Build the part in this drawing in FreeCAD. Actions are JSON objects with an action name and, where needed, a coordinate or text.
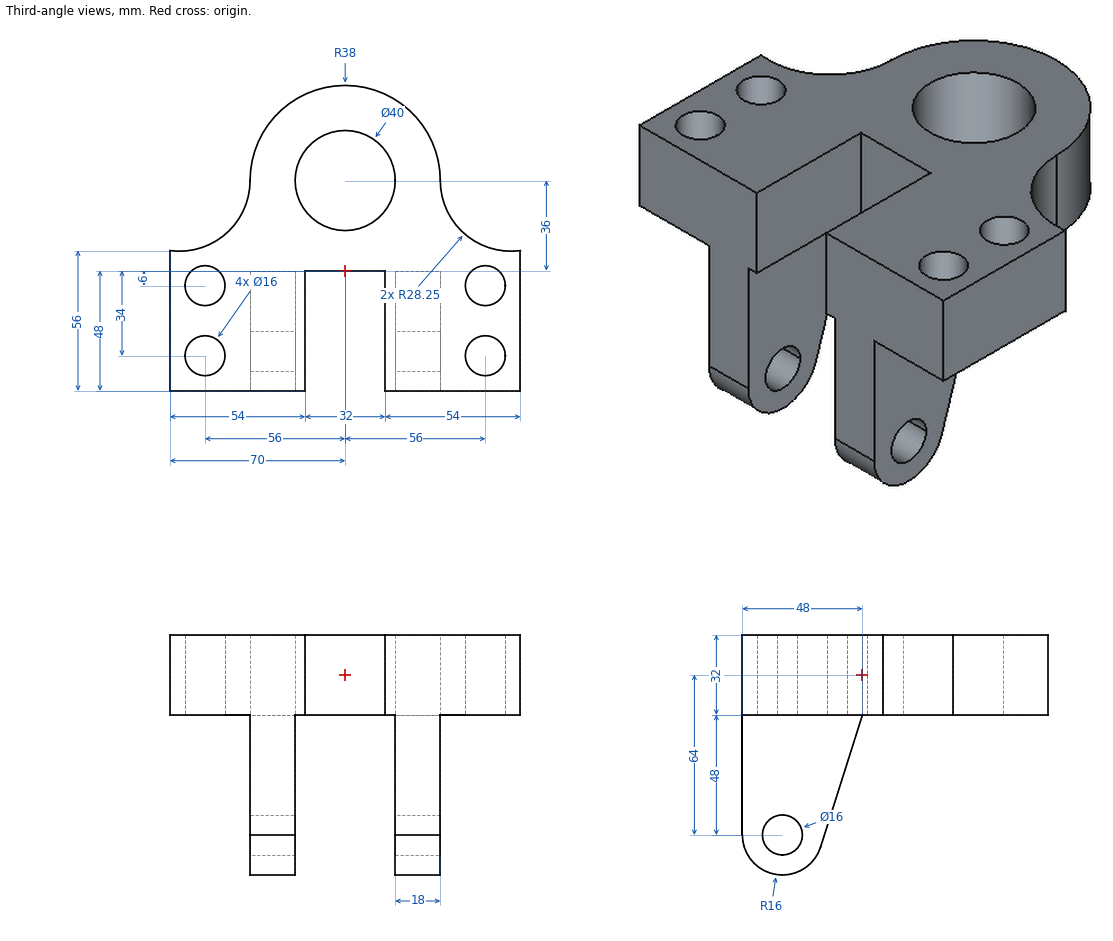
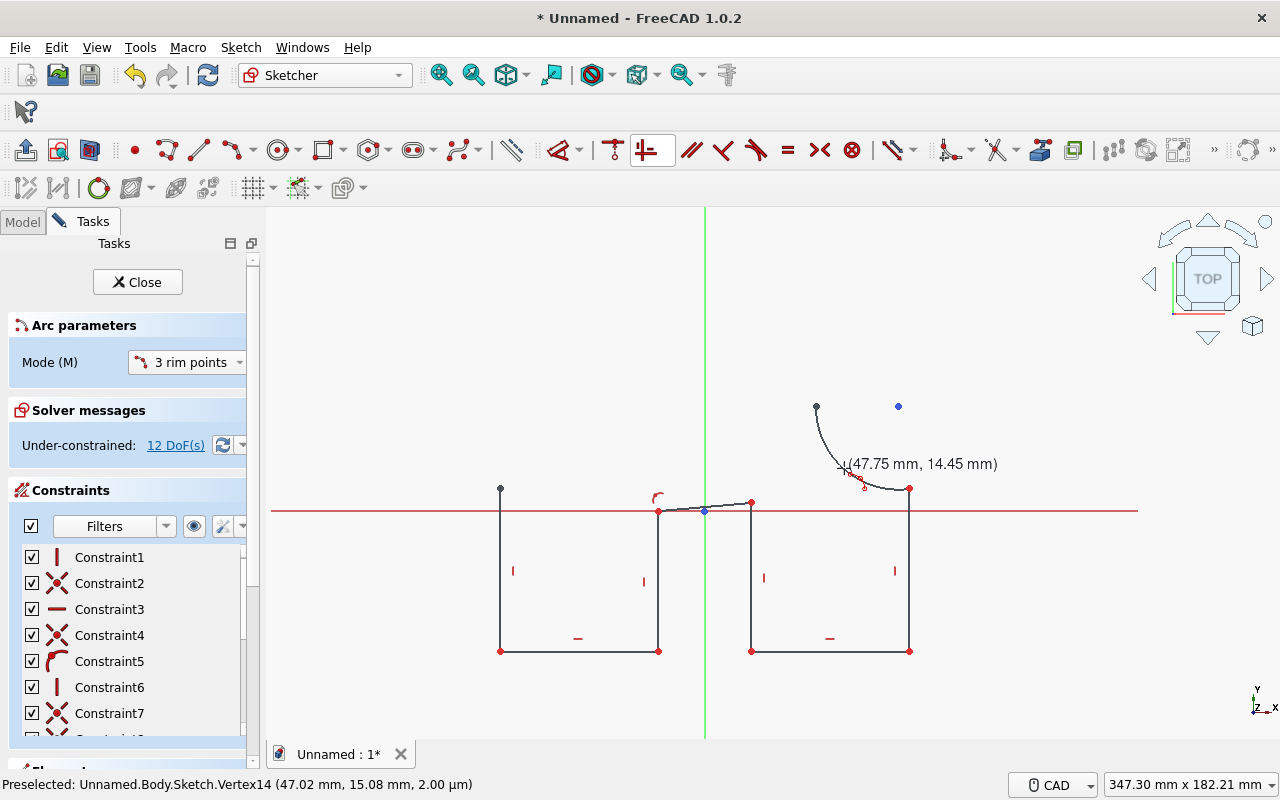
{"action": "left_click", "coordinate": [816, 407]}
{"action": "left_click", "coordinate": [594, 406]}
{"action": "left_click", "coordinate": [739, 301]}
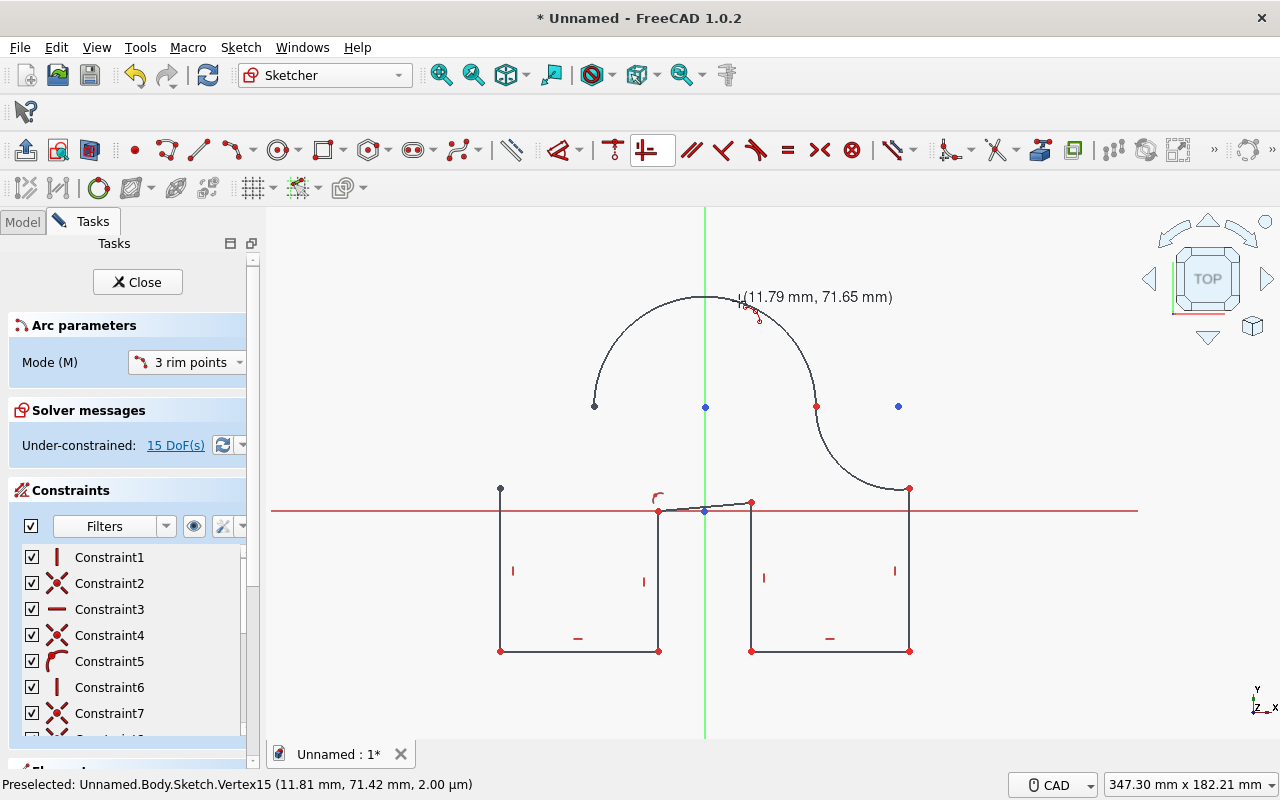
{"action": "left_click", "coordinate": [594, 407]}
{"action": "left_click", "coordinate": [500, 489]}
{"action": "left_click", "coordinate": [565, 468]}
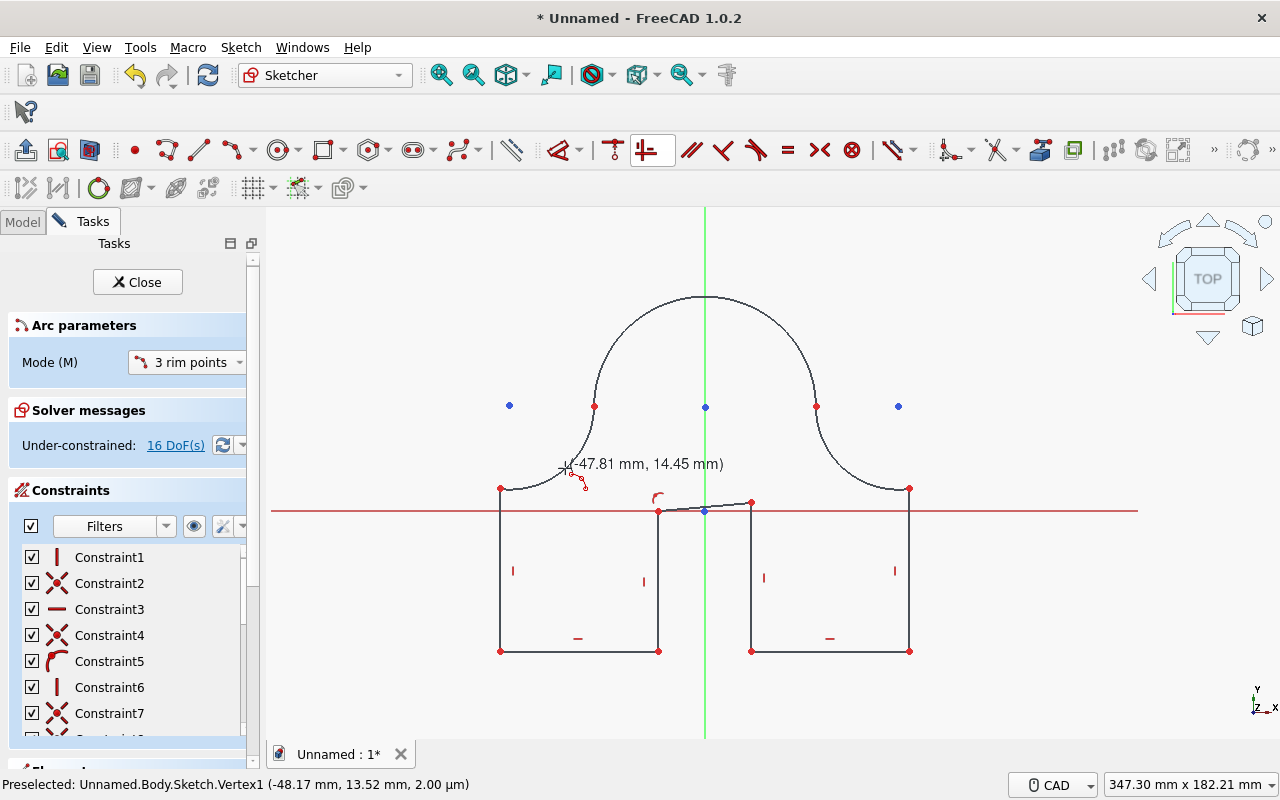
{"action": "left_click", "coordinate": [278, 150]}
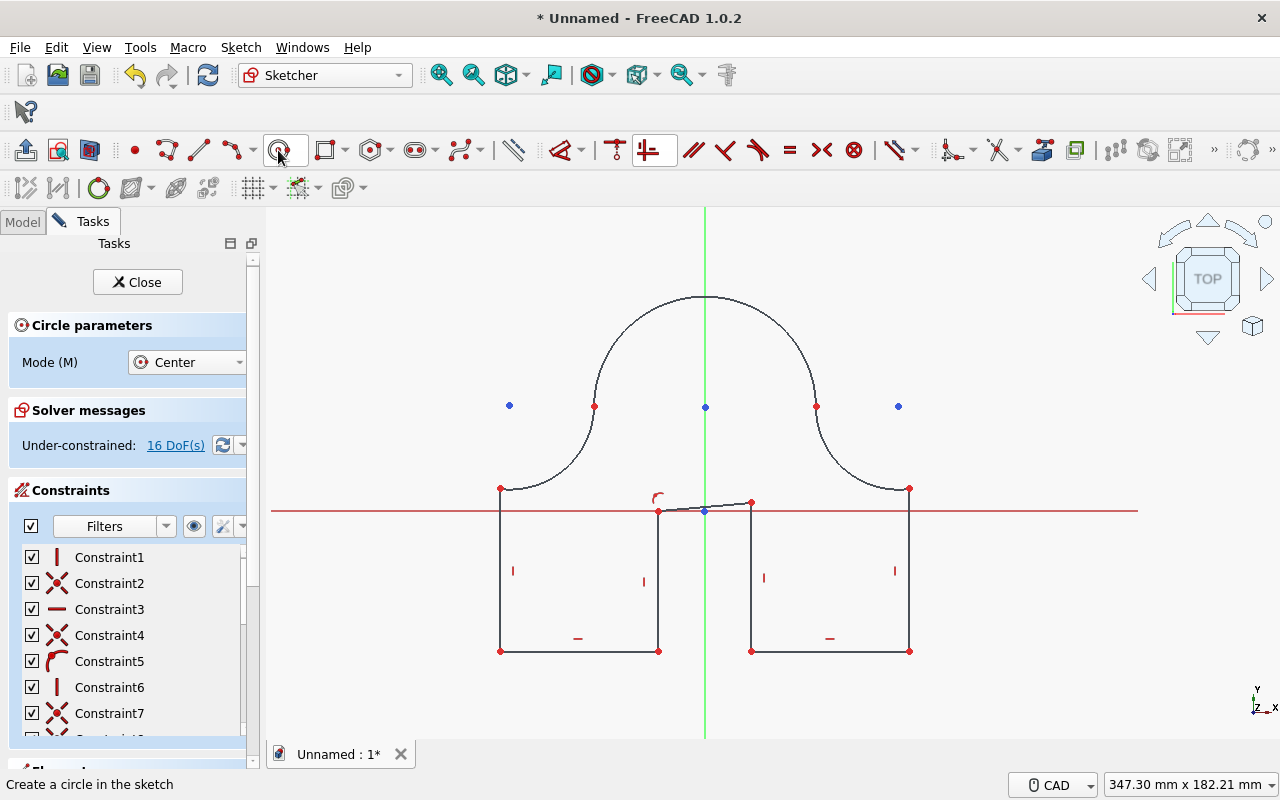
{"action": "left_click", "coordinate": [541, 610]}
{"action": "mouse_move", "coordinate": [558, 594]}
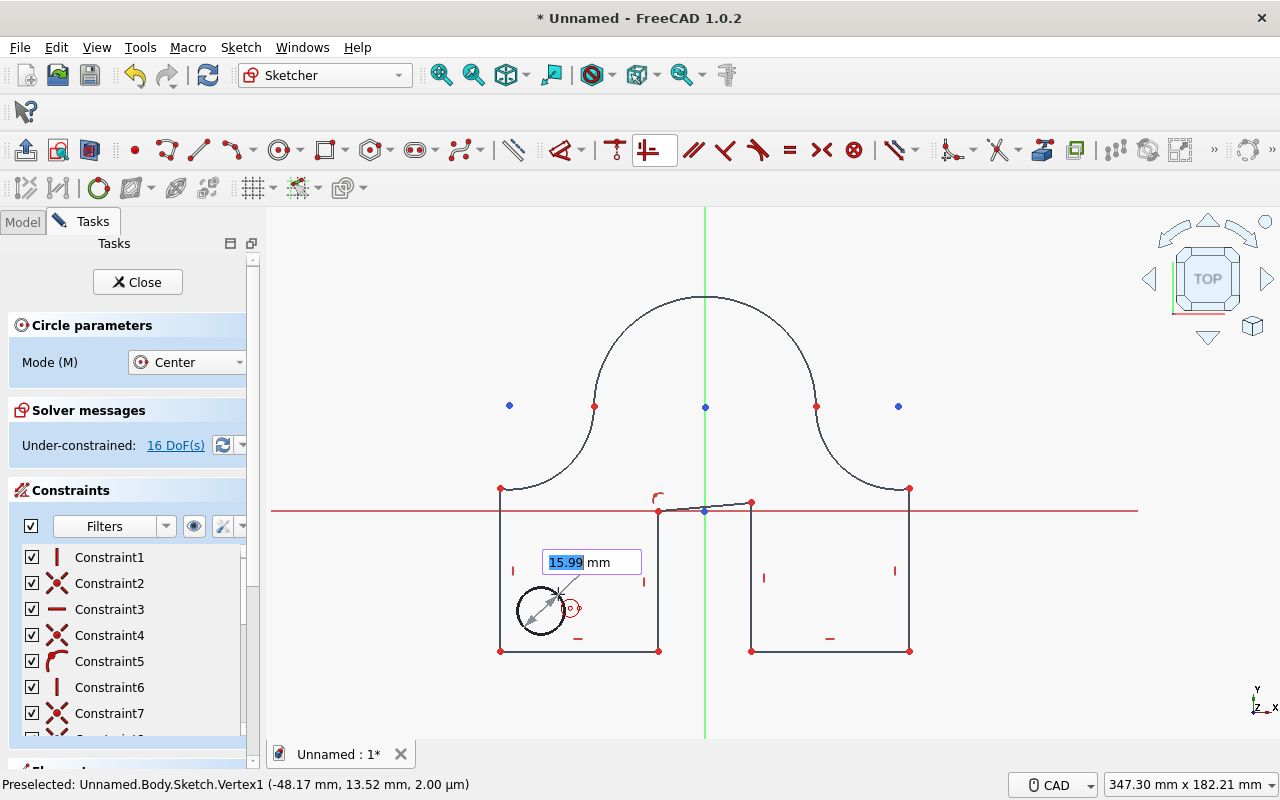
{"action": "type", "text": "16"}
{"action": "key", "text": "Return"}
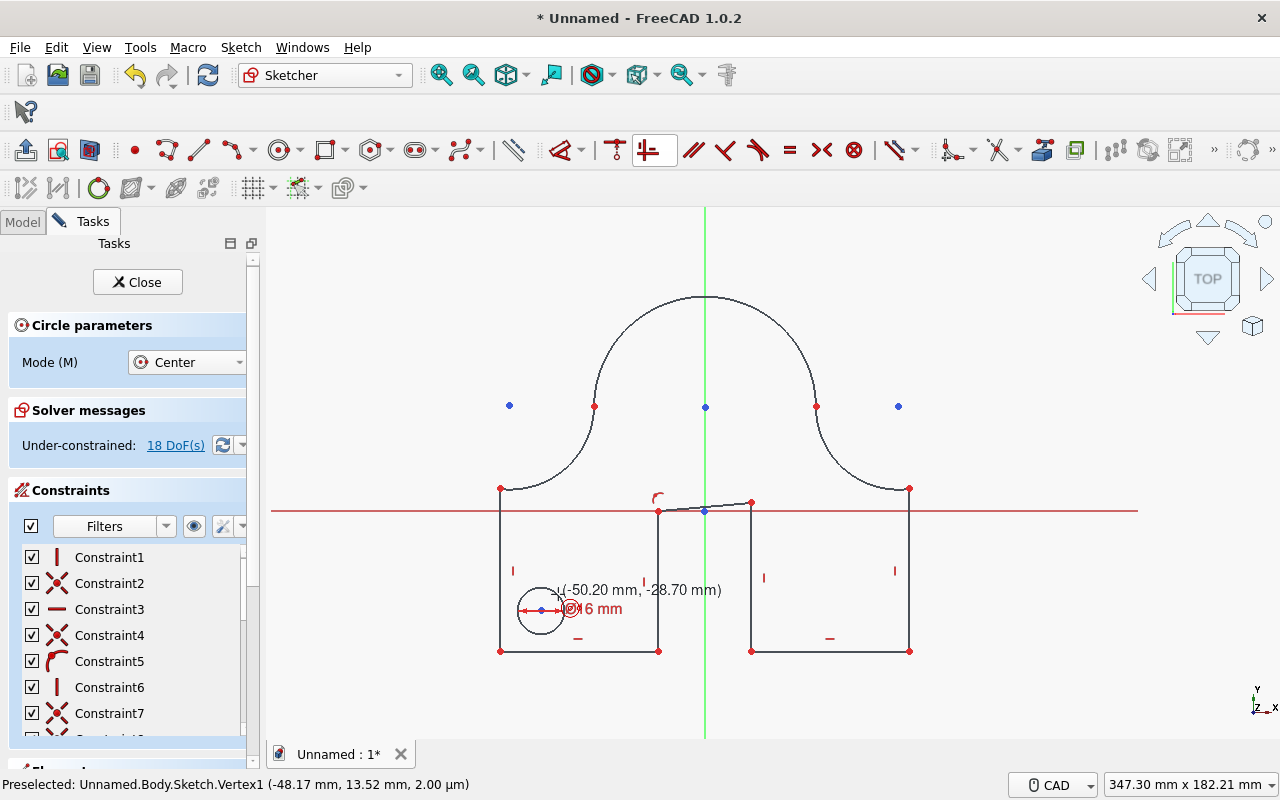
{"action": "left_click", "coordinate": [541, 529]}
{"action": "mouse_move", "coordinate": [558, 545]}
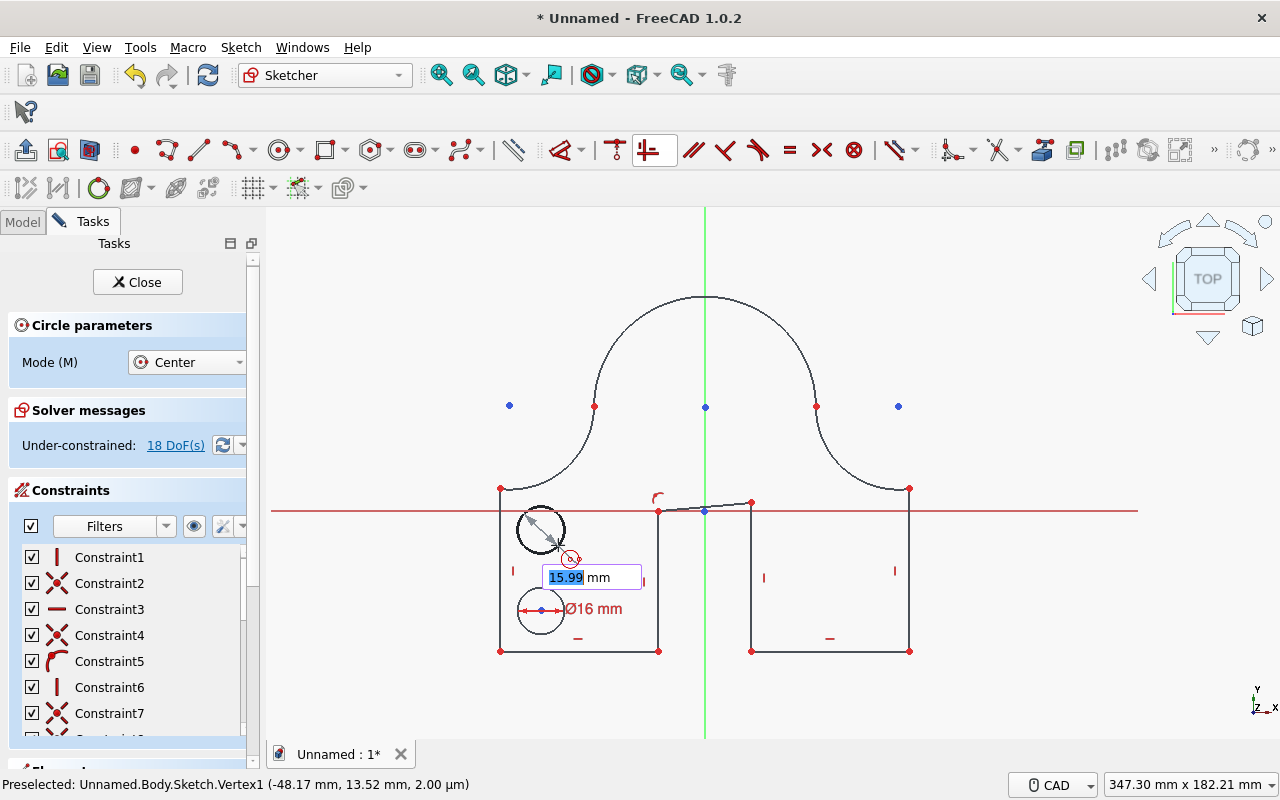
{"action": "type", "text": "16"}
{"action": "key", "text": "Return"}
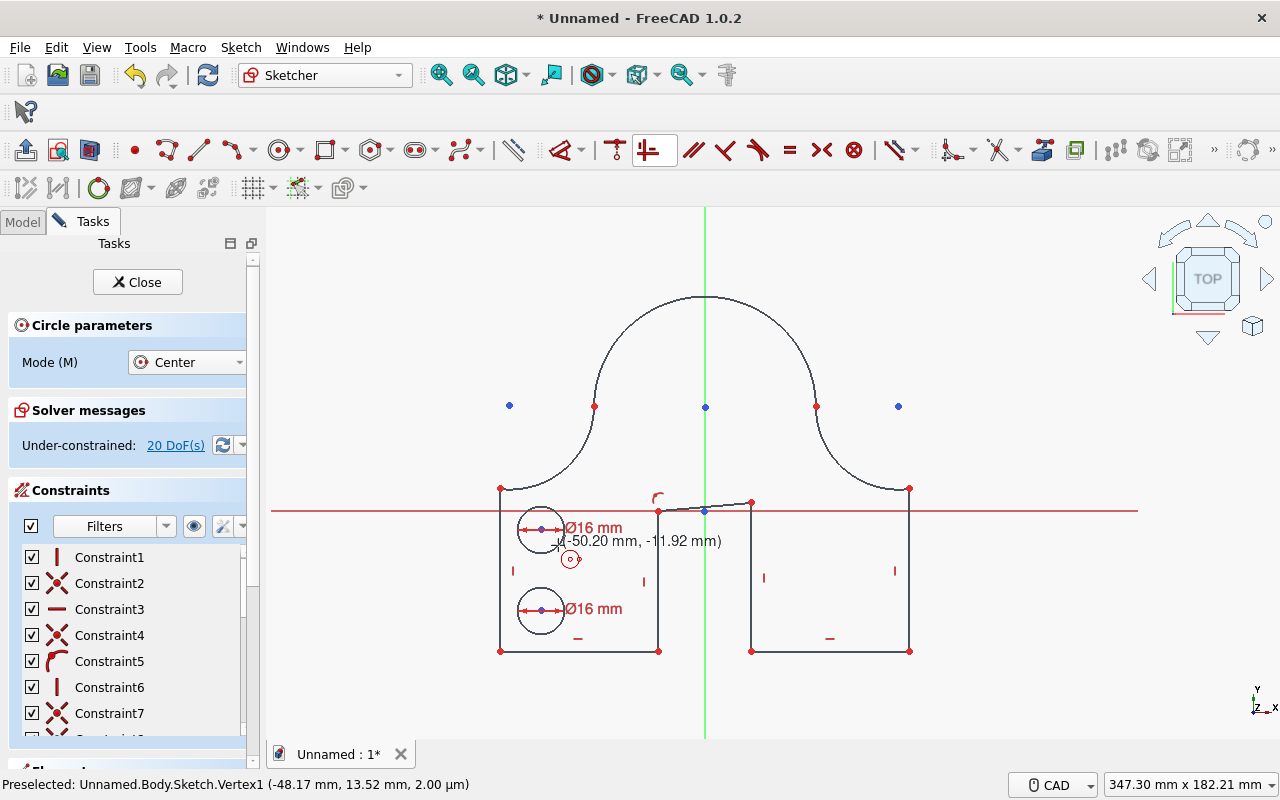
{"action": "left_click", "coordinate": [868, 610]}
{"action": "mouse_move", "coordinate": [885, 594]}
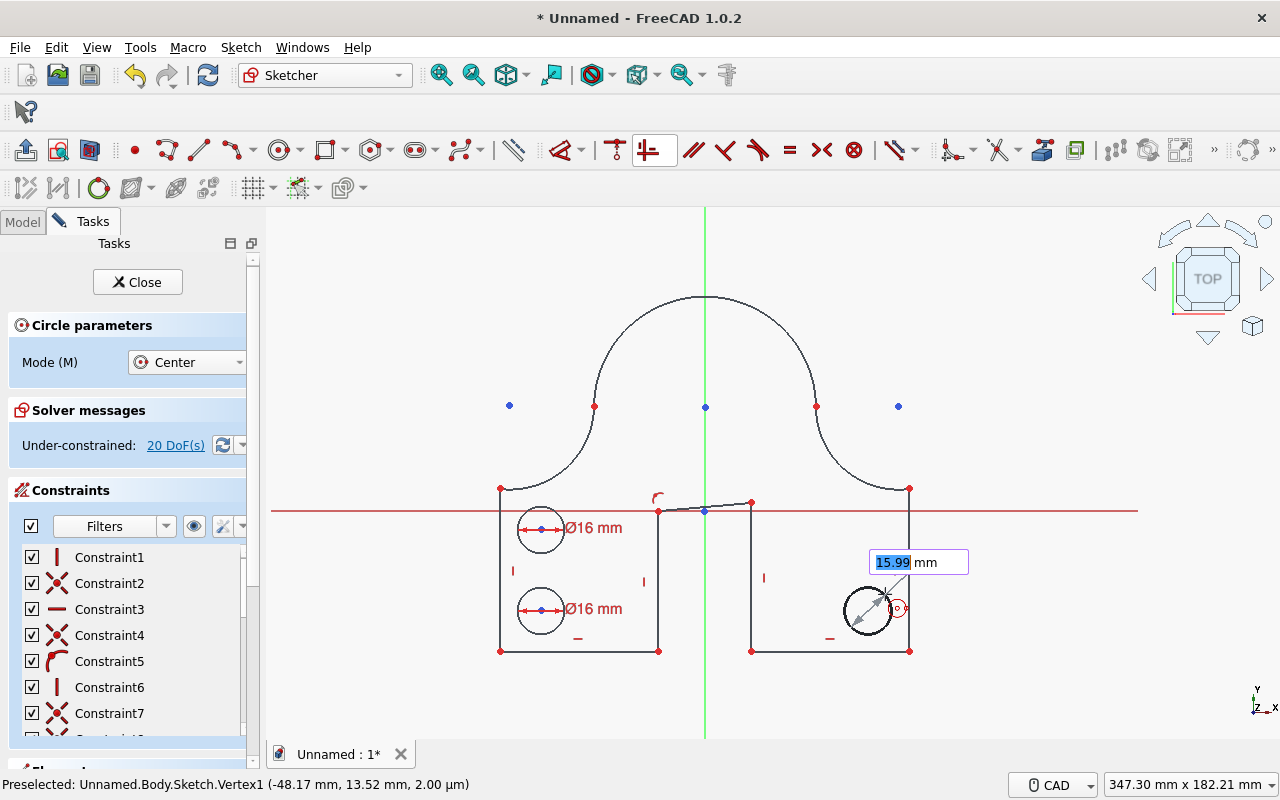
{"action": "type", "text": "16"}
{"action": "key", "text": "Return"}